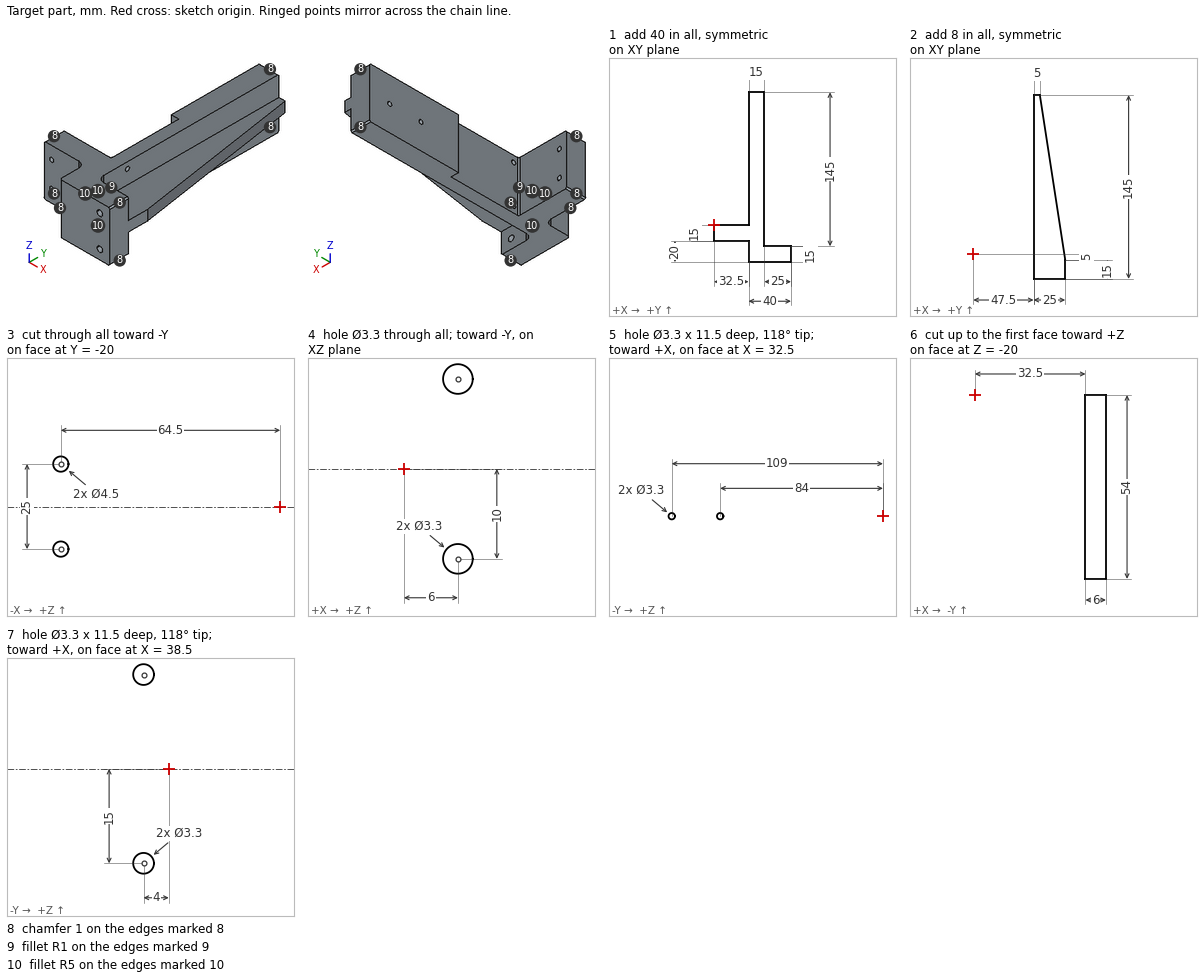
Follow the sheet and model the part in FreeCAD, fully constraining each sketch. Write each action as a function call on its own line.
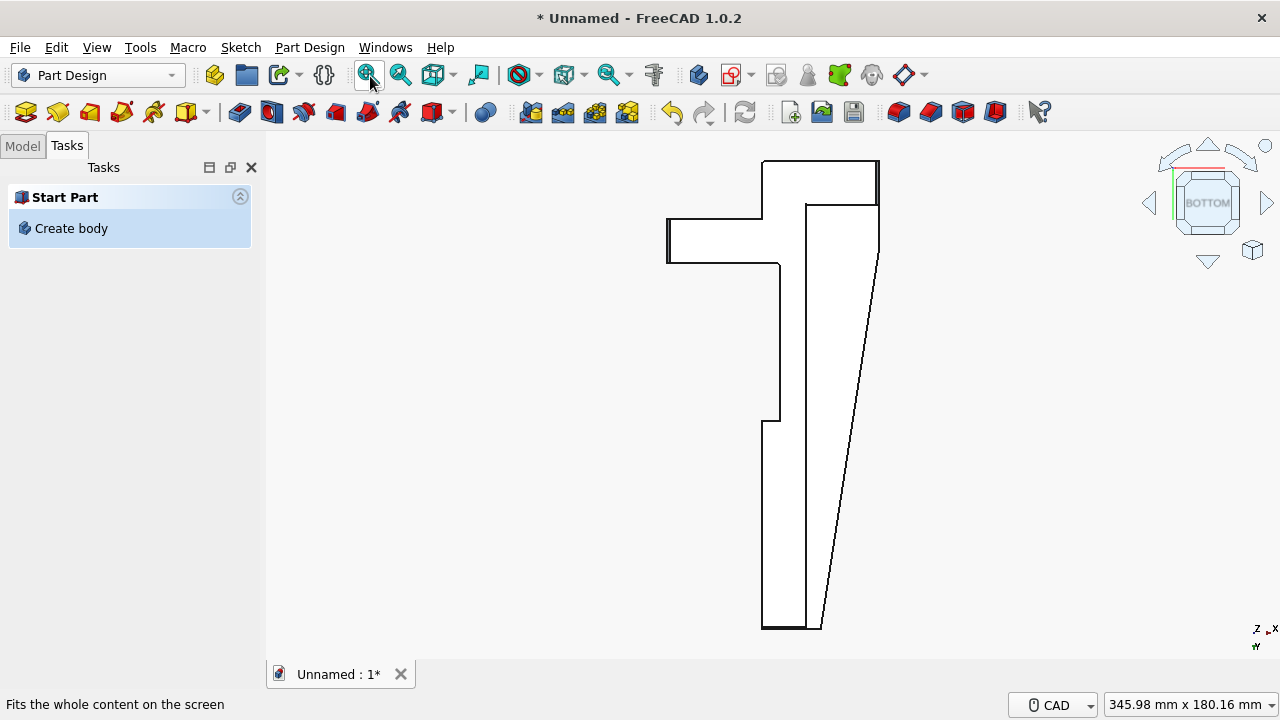
key(4)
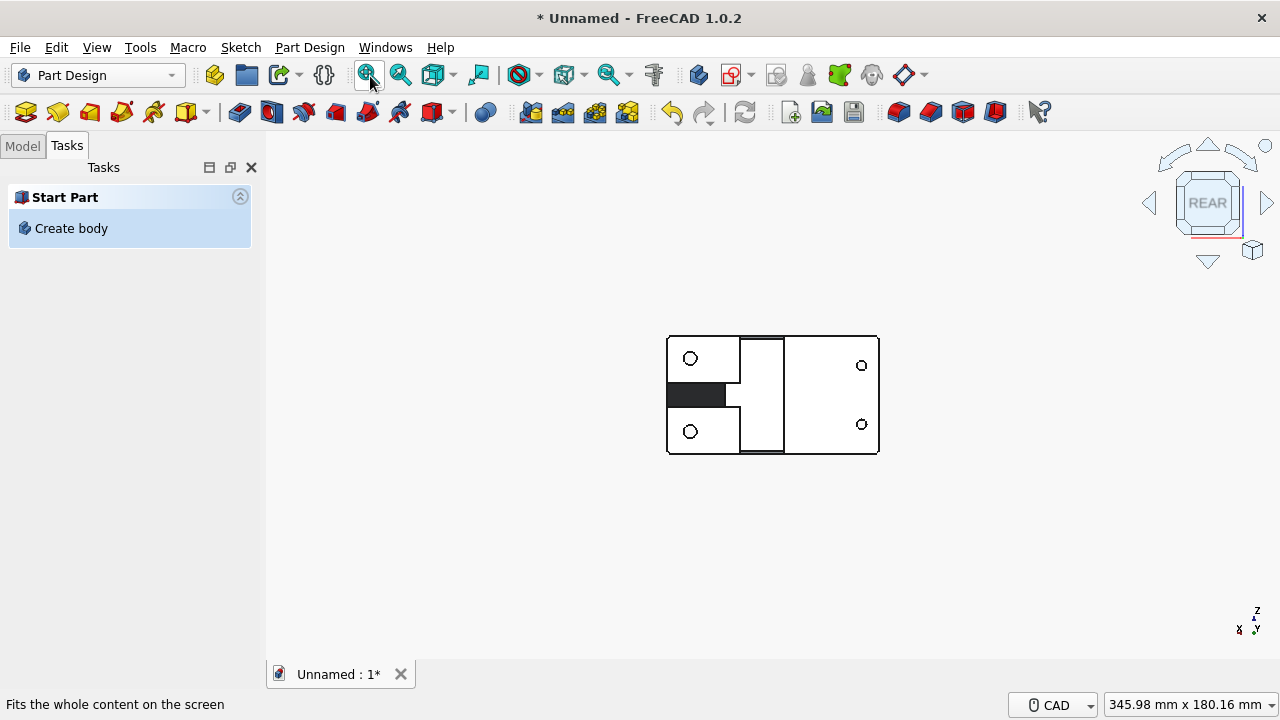
click(370, 76)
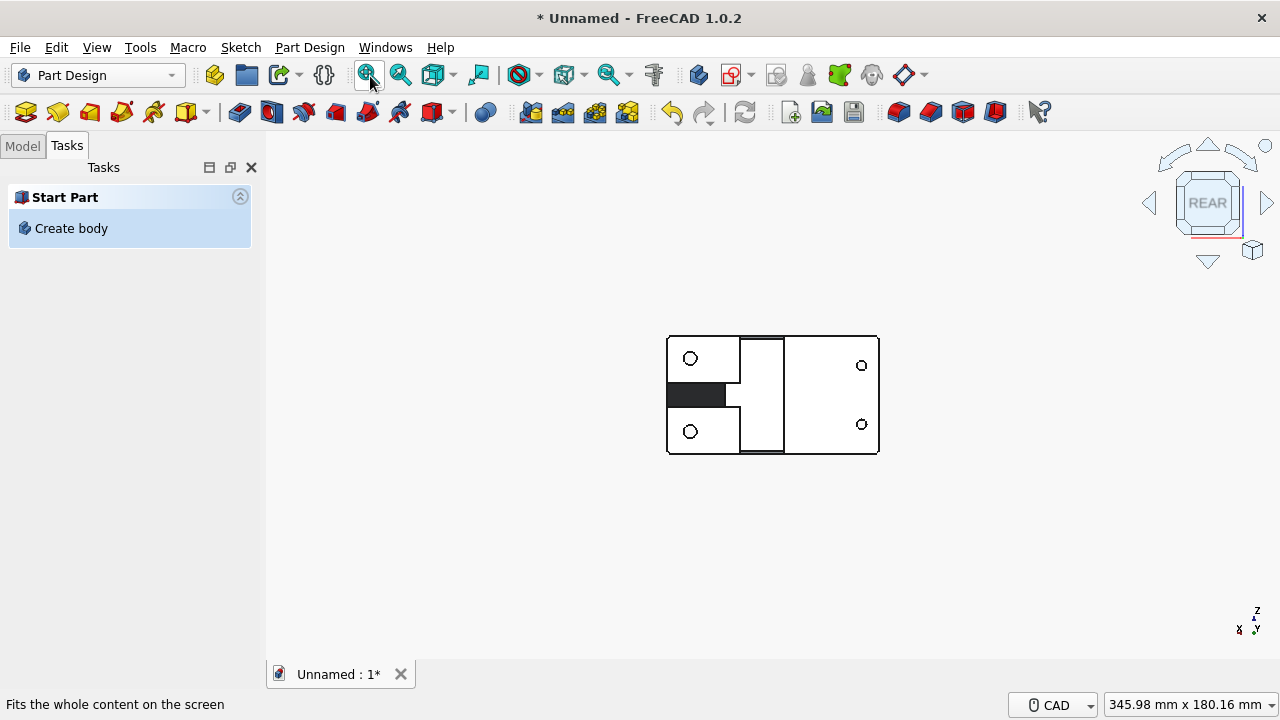
key(6)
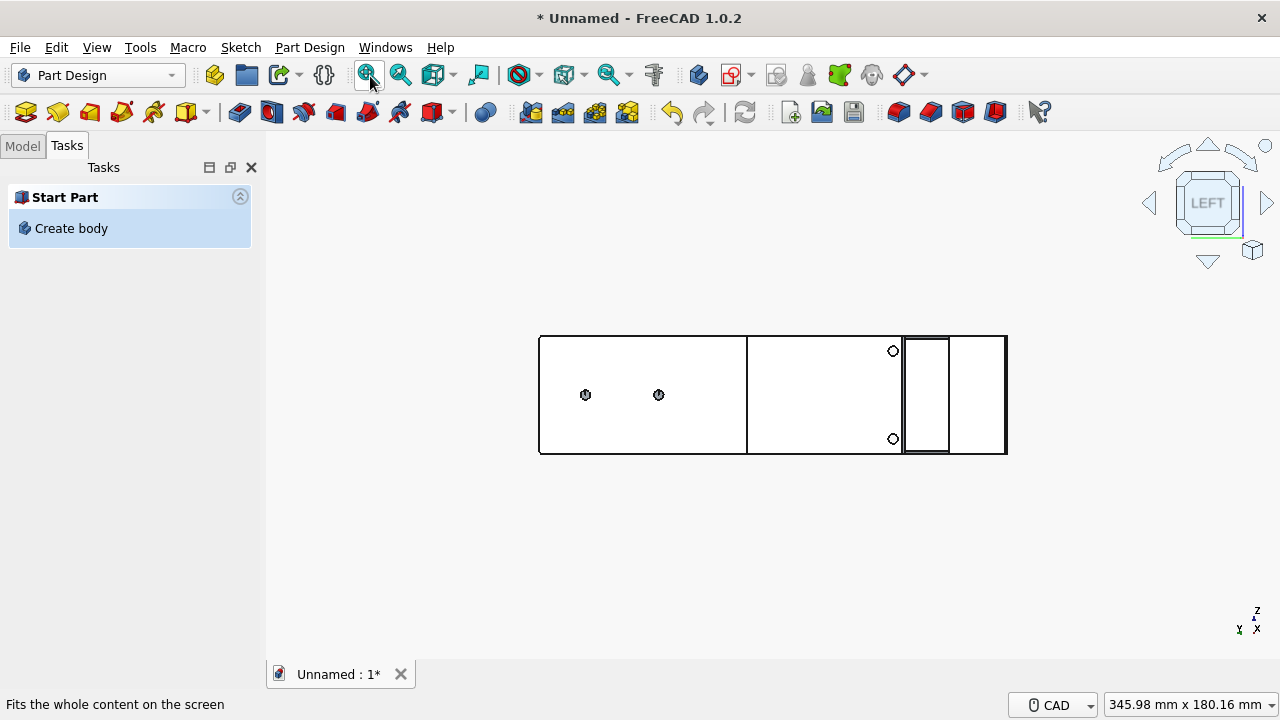
key(v)
key(3)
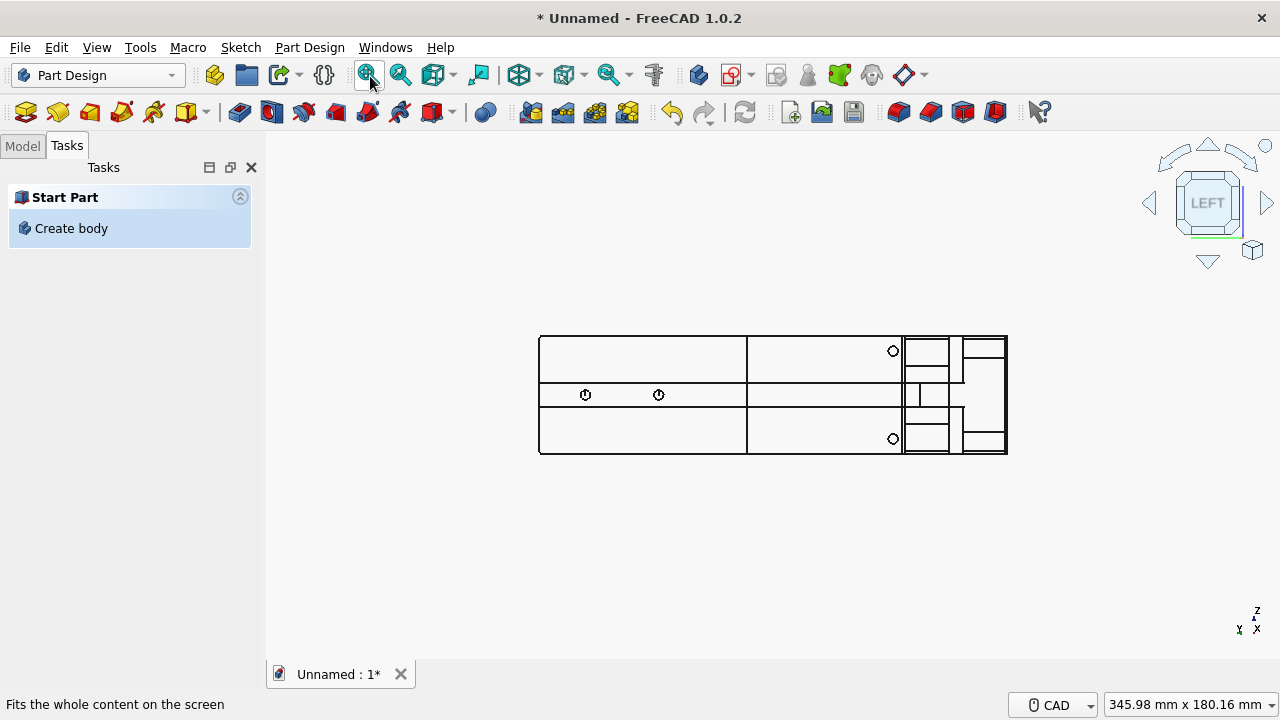
key(0)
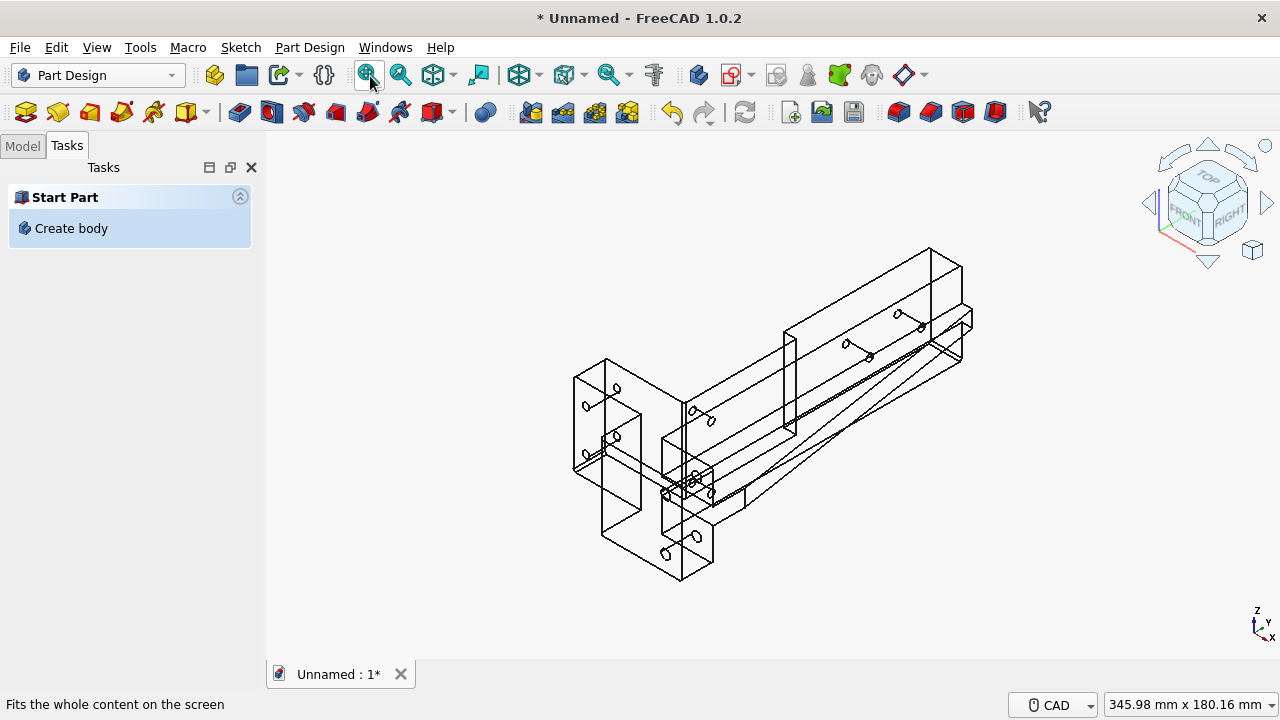
click(662, 457)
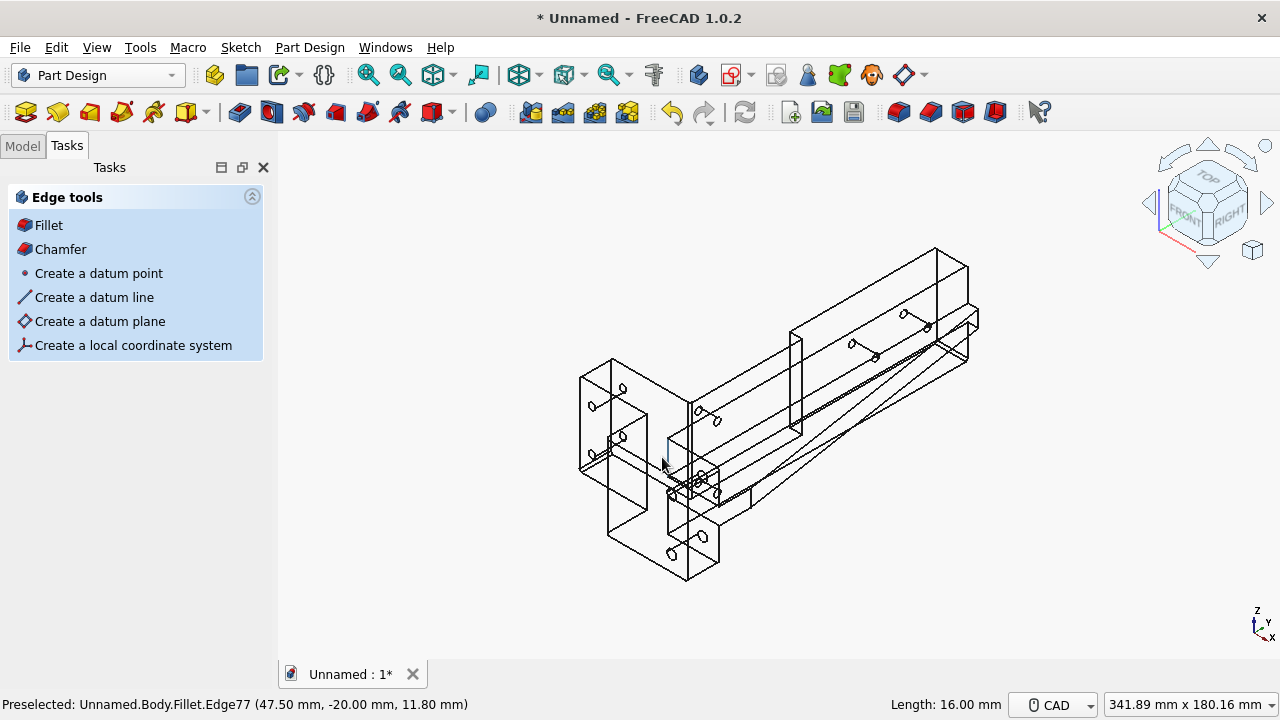
click(647, 471, ctrl)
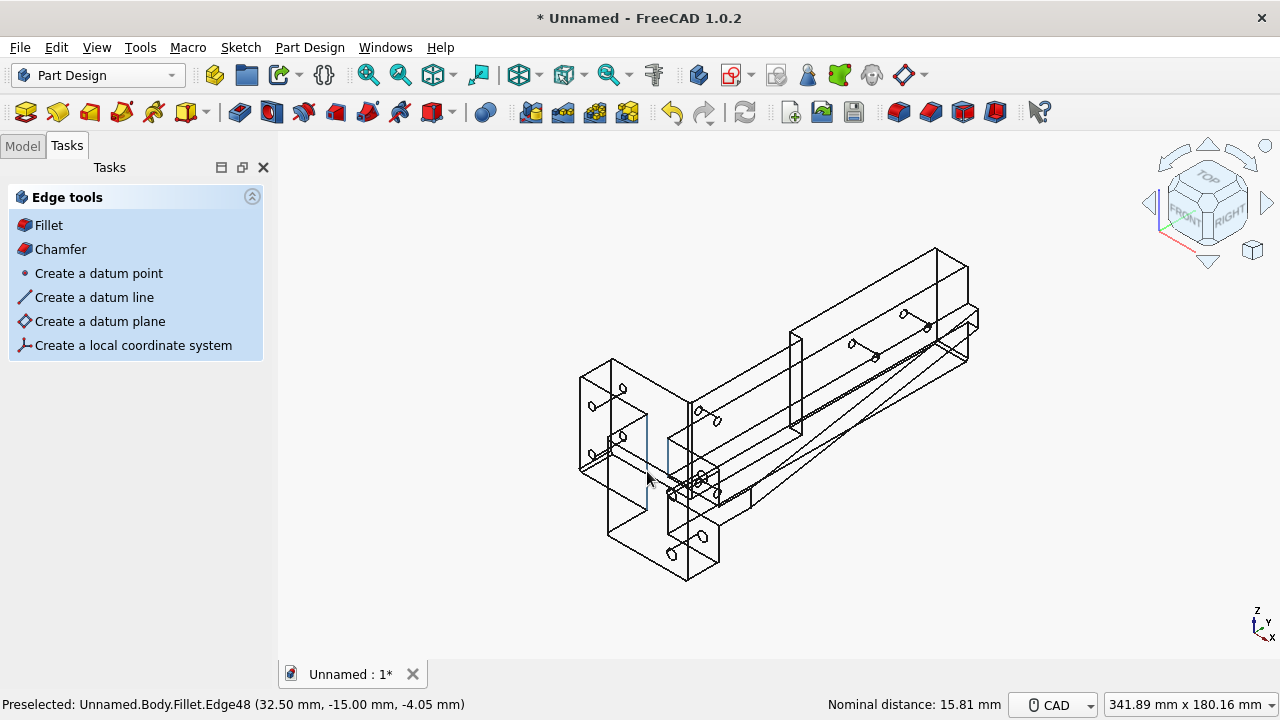
click(668, 514, ctrl)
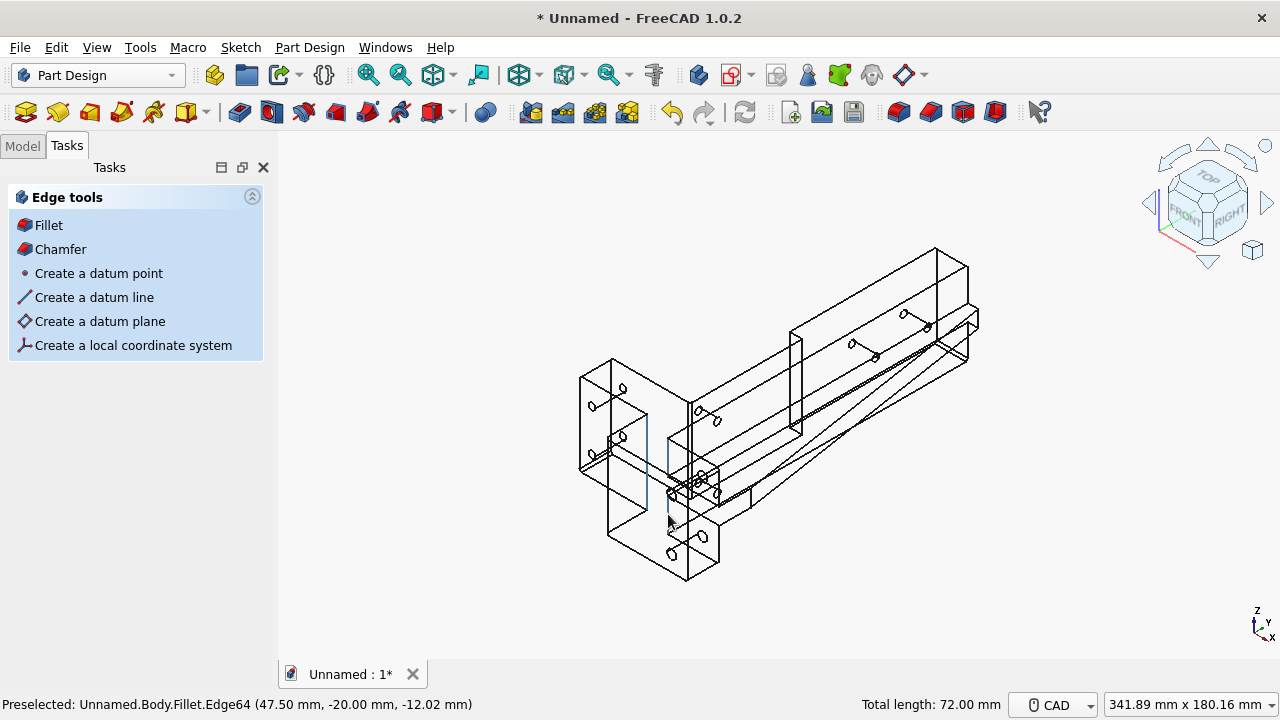
key(v)
key(1)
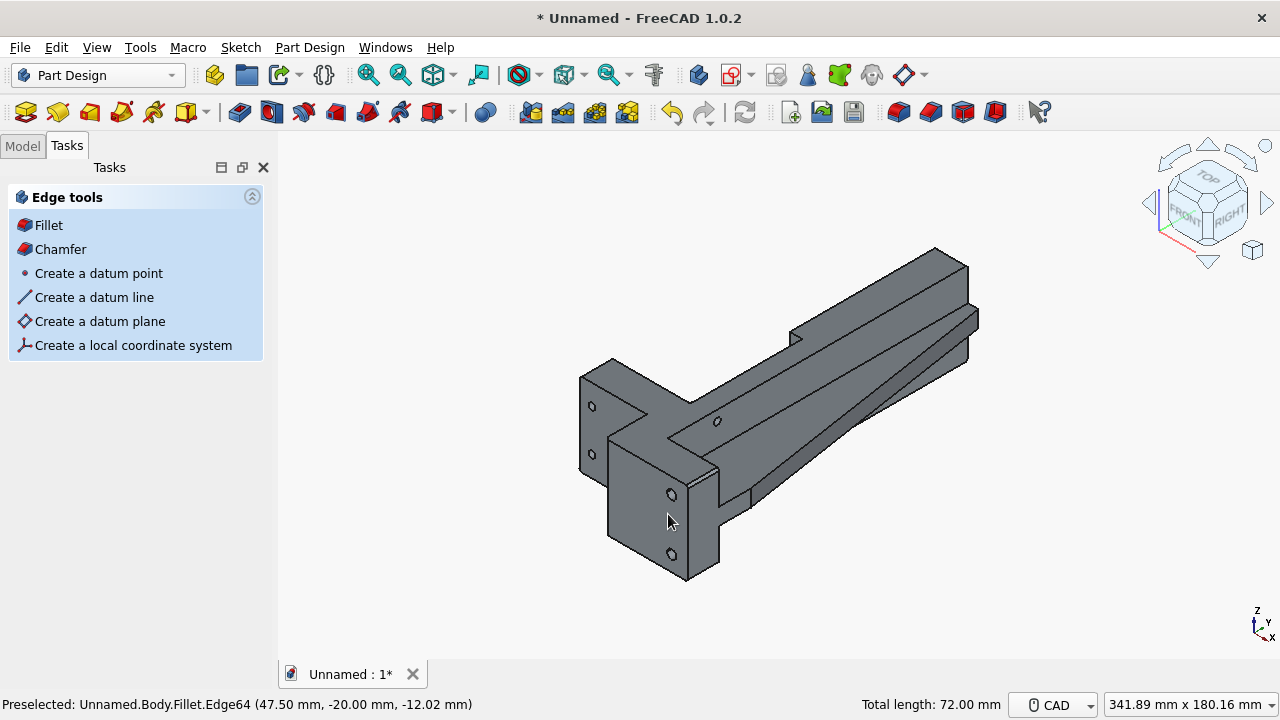
click(900, 112)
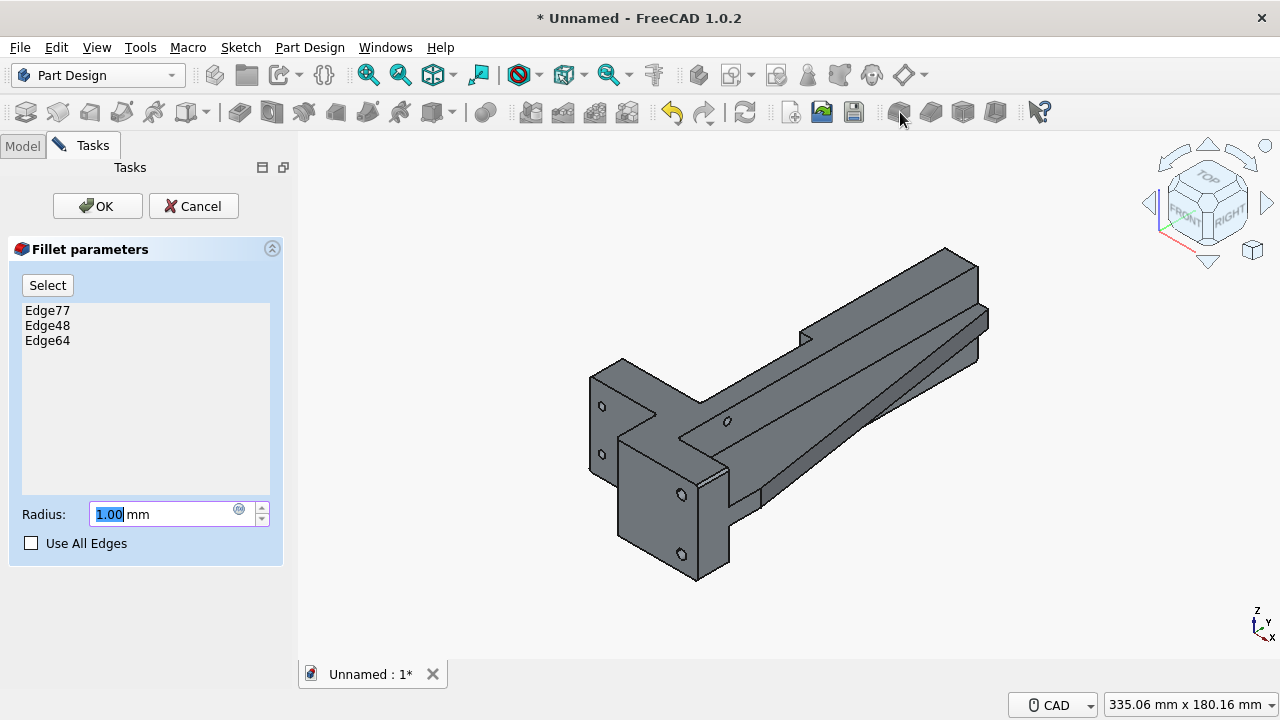
text(5)
key(Tab)